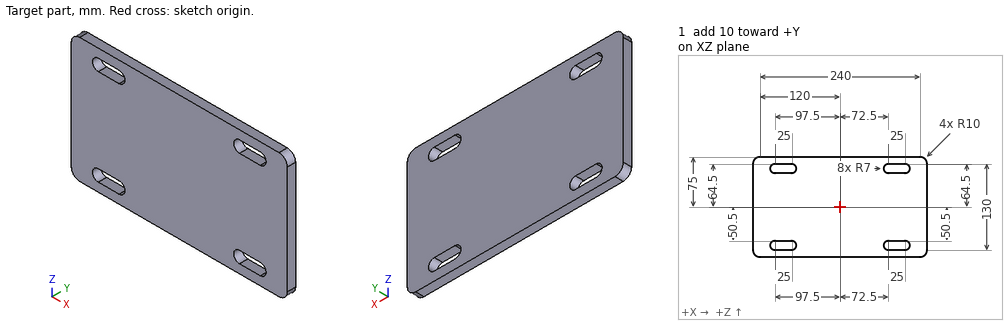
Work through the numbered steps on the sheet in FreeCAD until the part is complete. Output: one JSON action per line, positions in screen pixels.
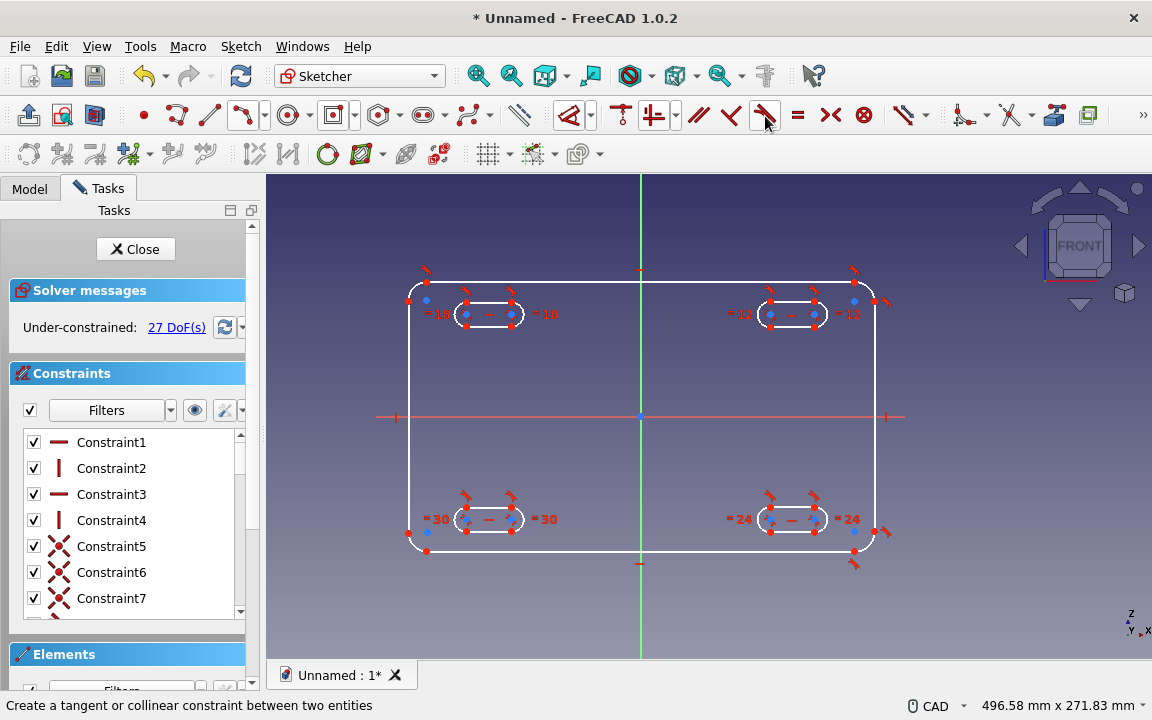
{"action": "left_click", "coordinate": [726, 552]}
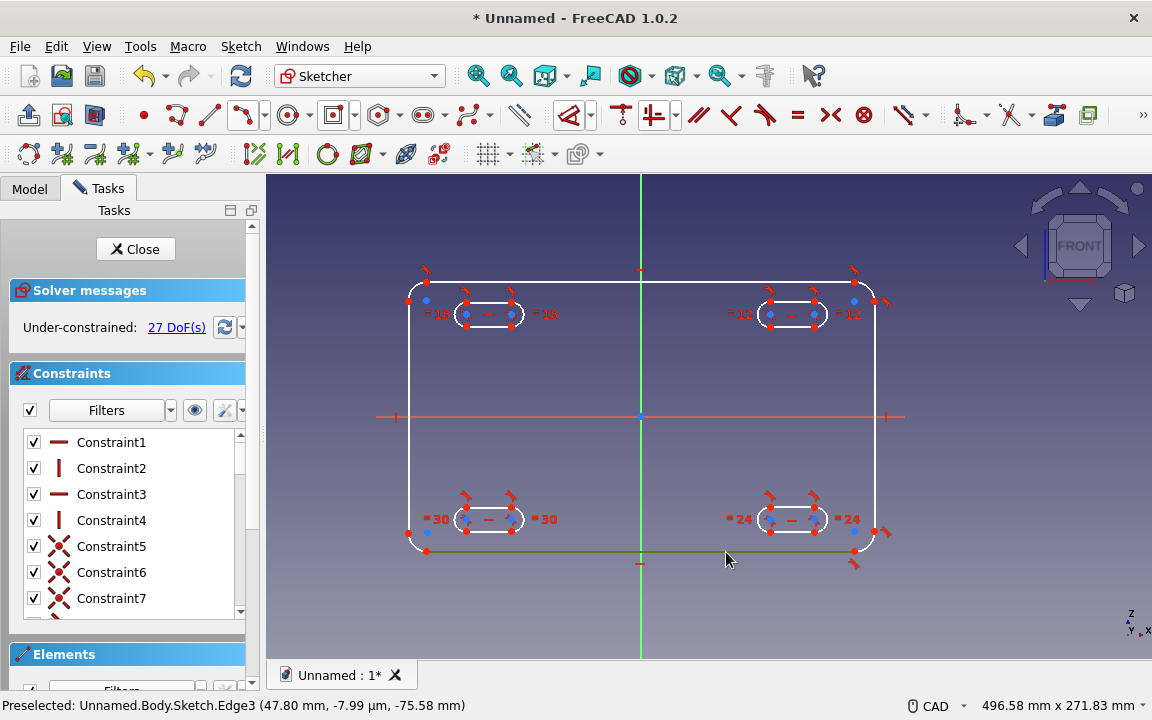
{"action": "left_click", "coordinate": [414, 546]}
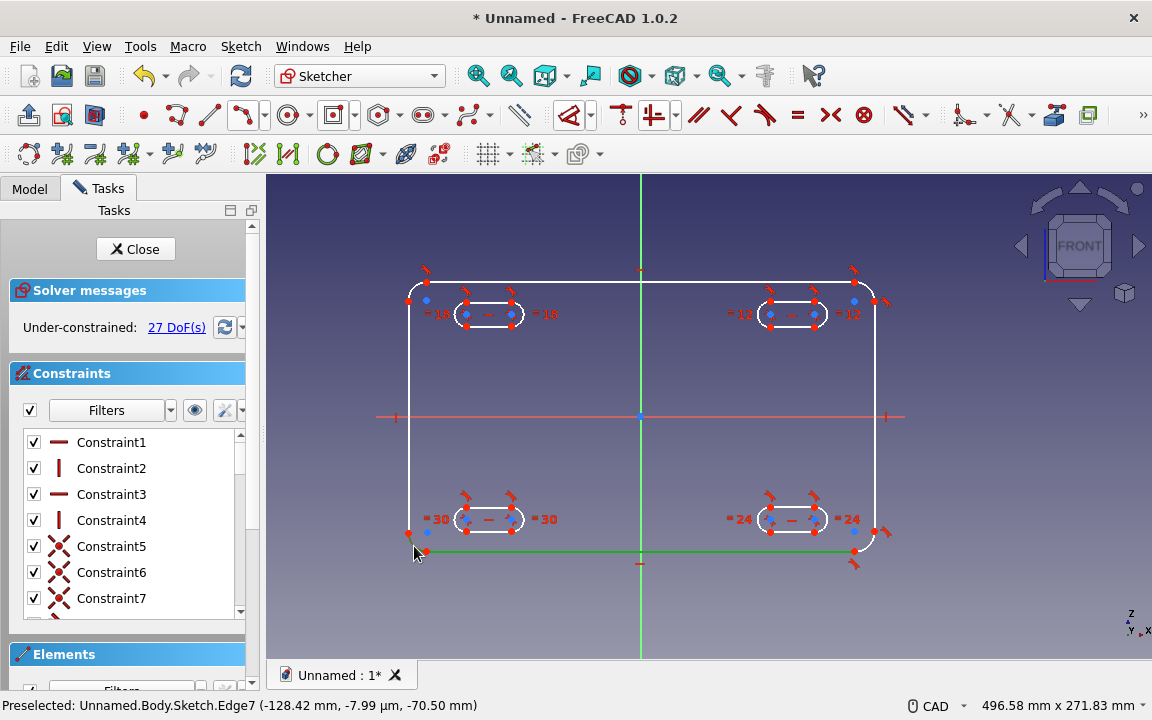
{"action": "left_click", "coordinate": [765, 116]}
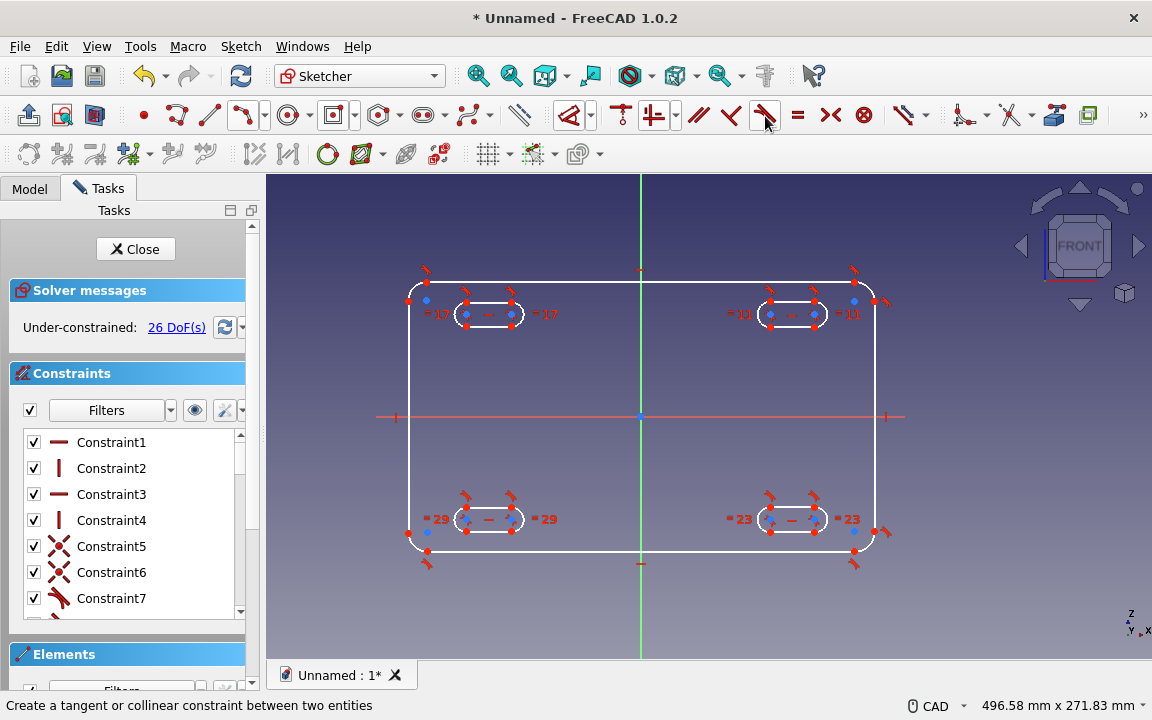
{"action": "left_click", "coordinate": [409, 464]}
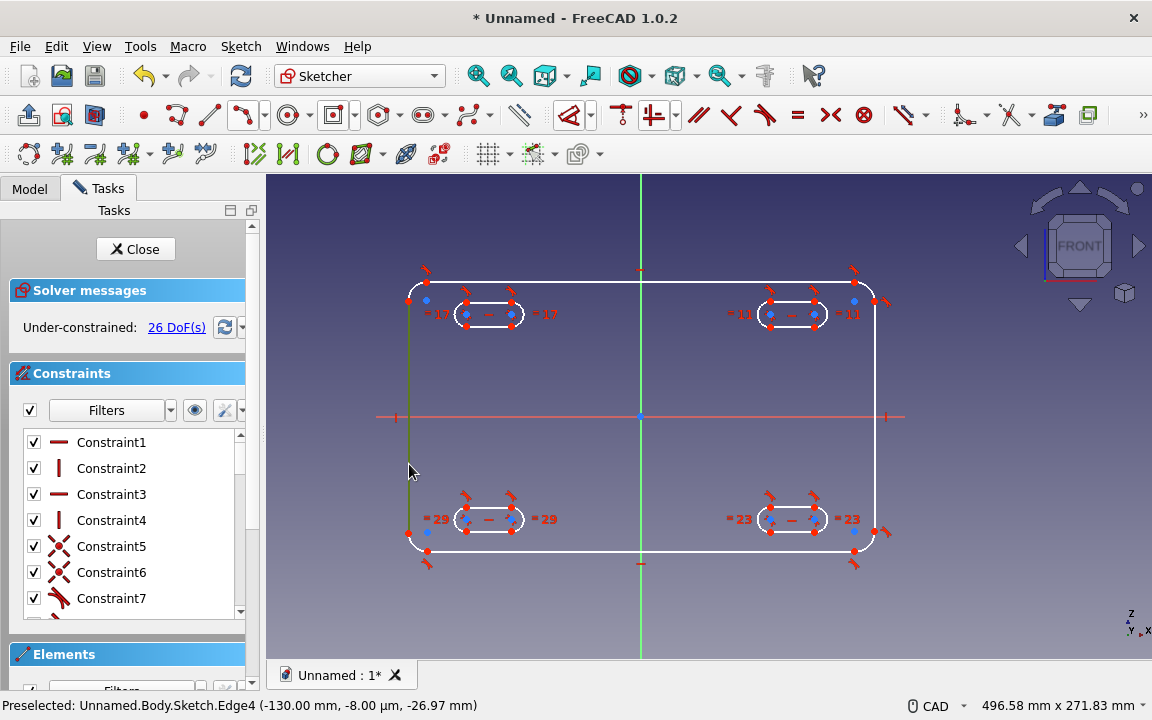
{"action": "left_click", "coordinate": [415, 547]}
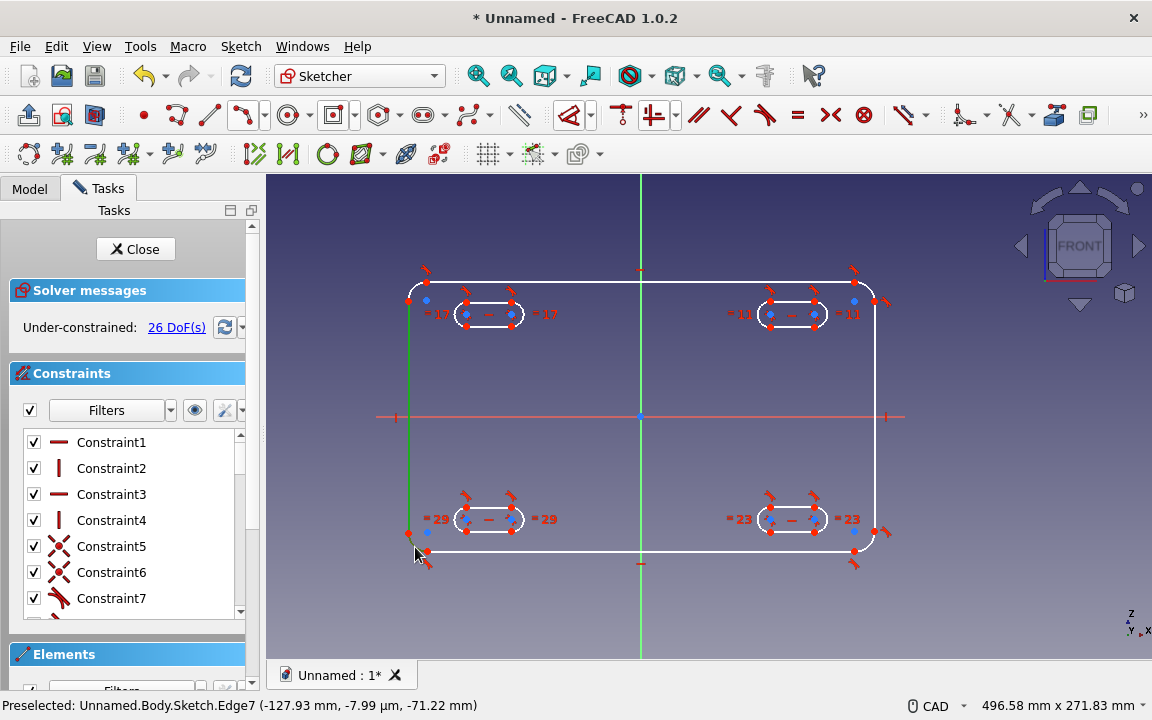
{"action": "left_click", "coordinate": [765, 116]}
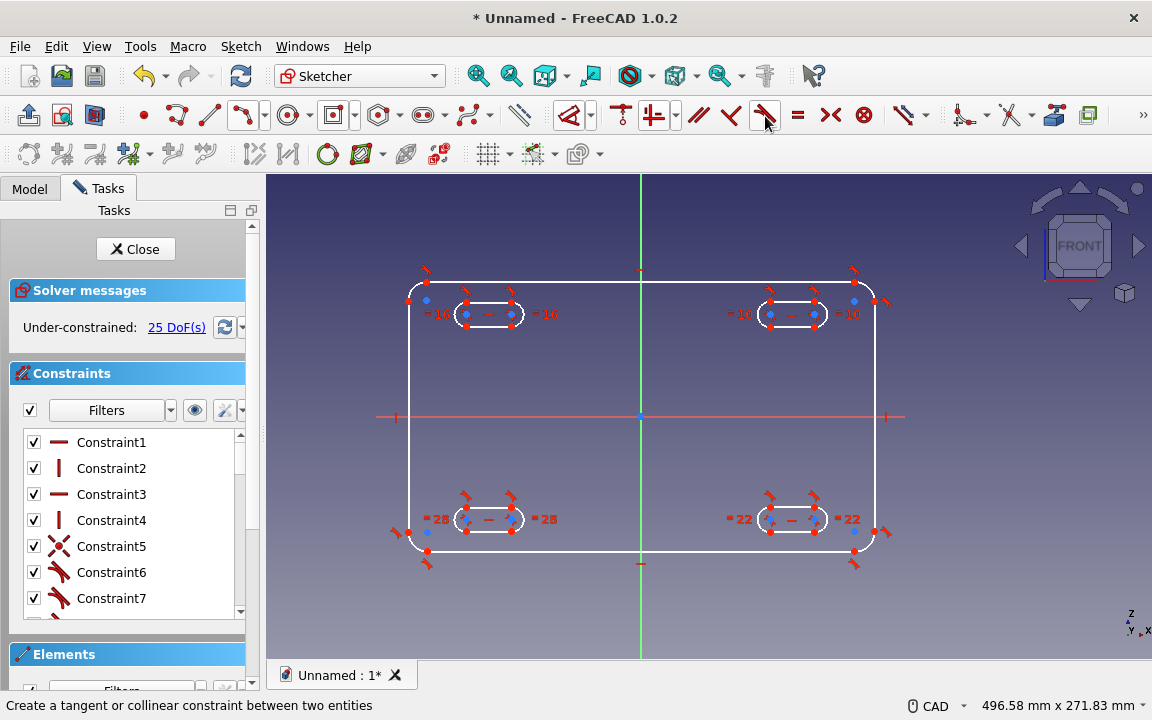
{"action": "left_click", "coordinate": [409, 463]}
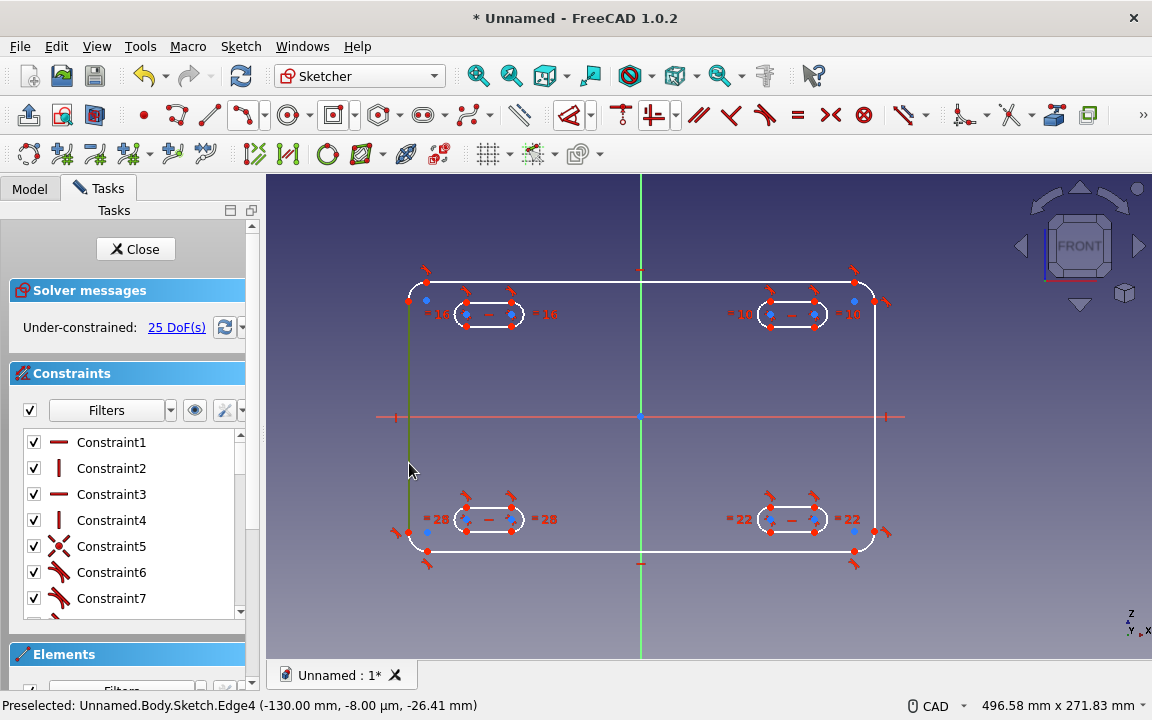
{"action": "left_click", "coordinate": [413, 288]}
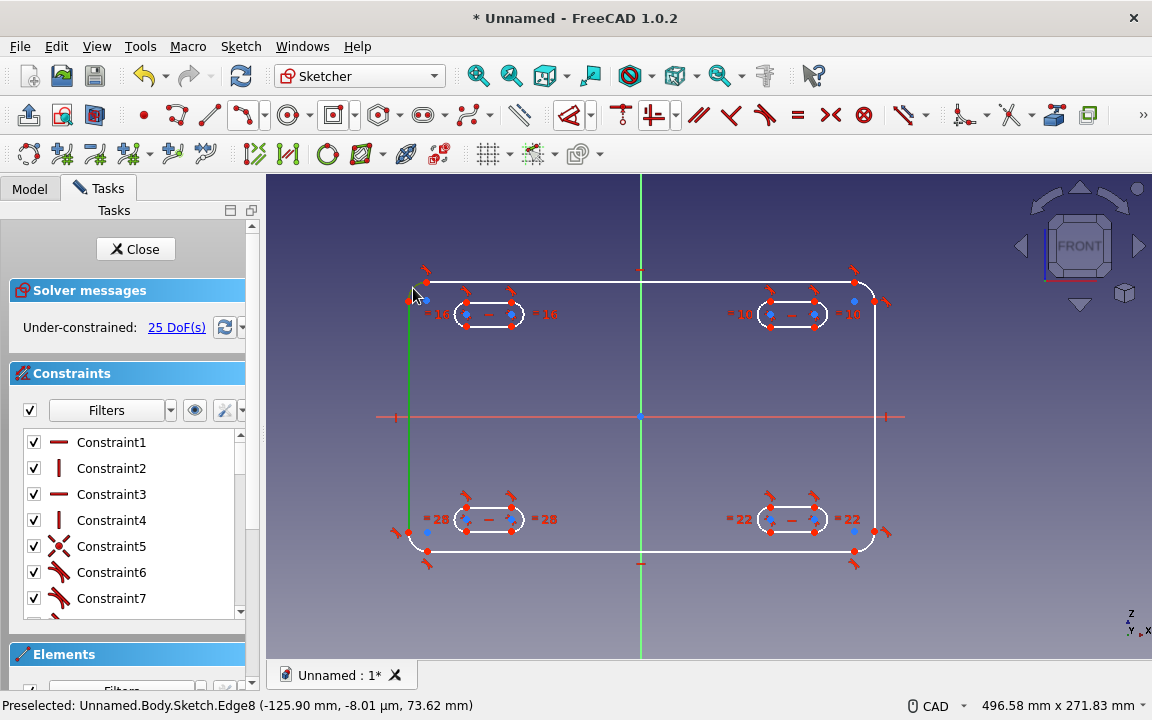
{"action": "left_click", "coordinate": [765, 116]}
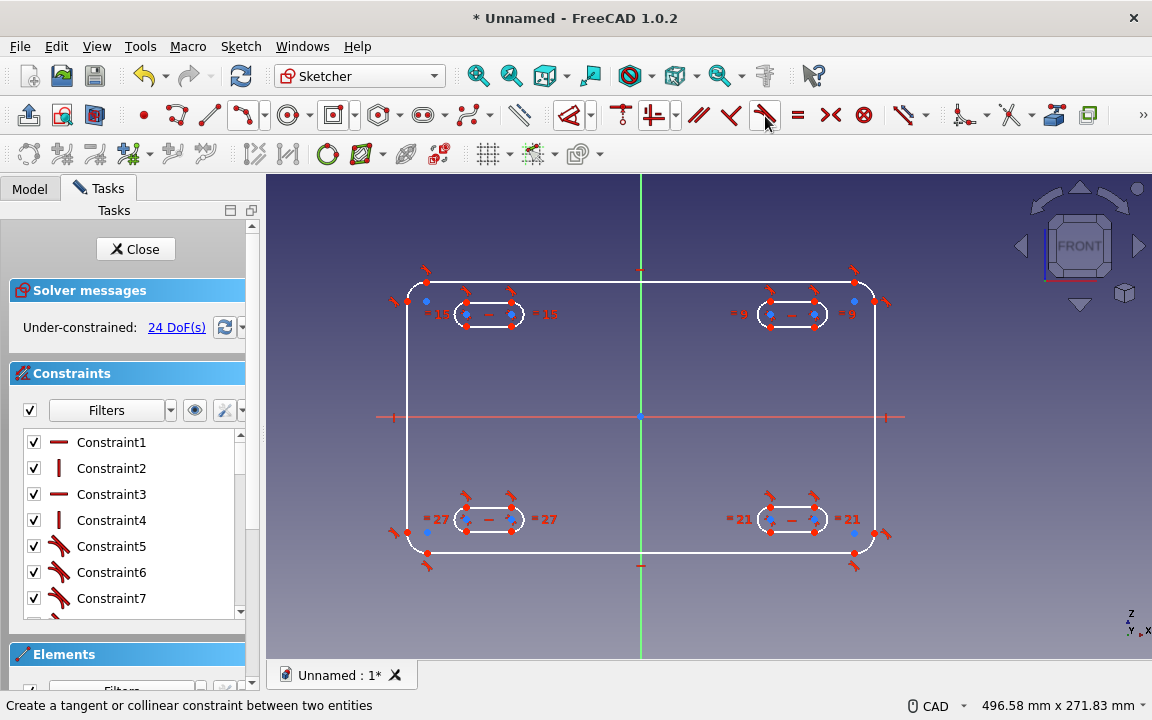
{"action": "scroll", "coordinate": [872, 293], "scroll_direction": "up", "scroll_amount": 3}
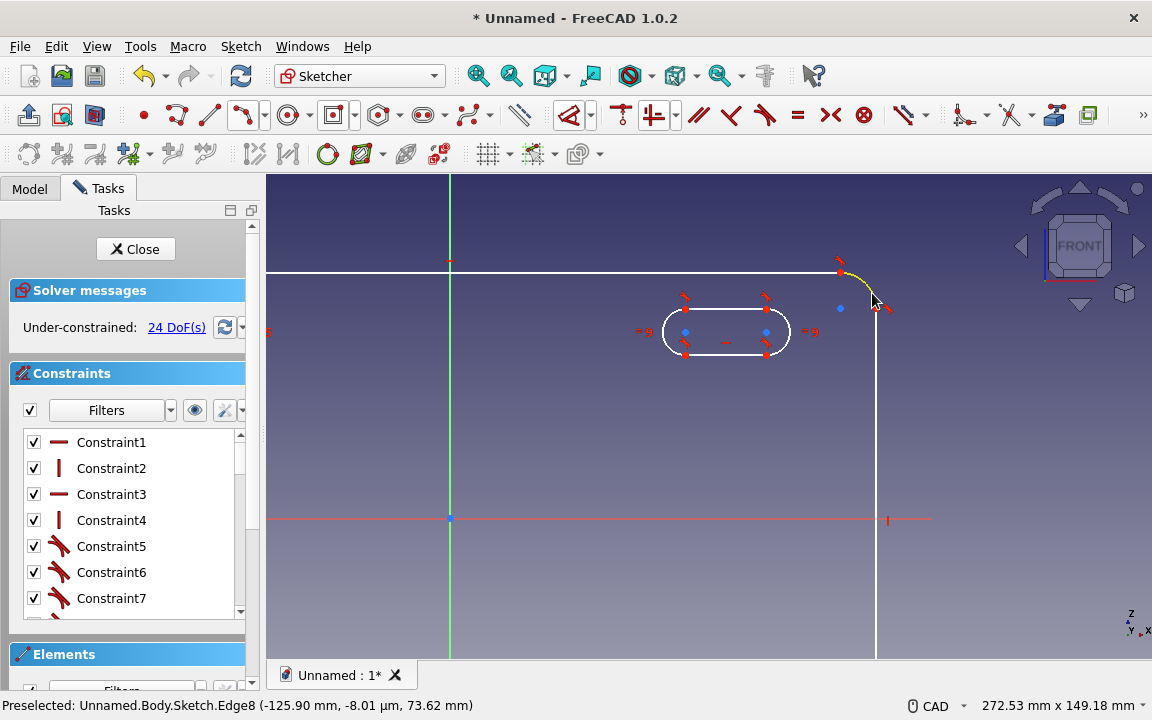
{"action": "left_click", "coordinate": [872, 293]}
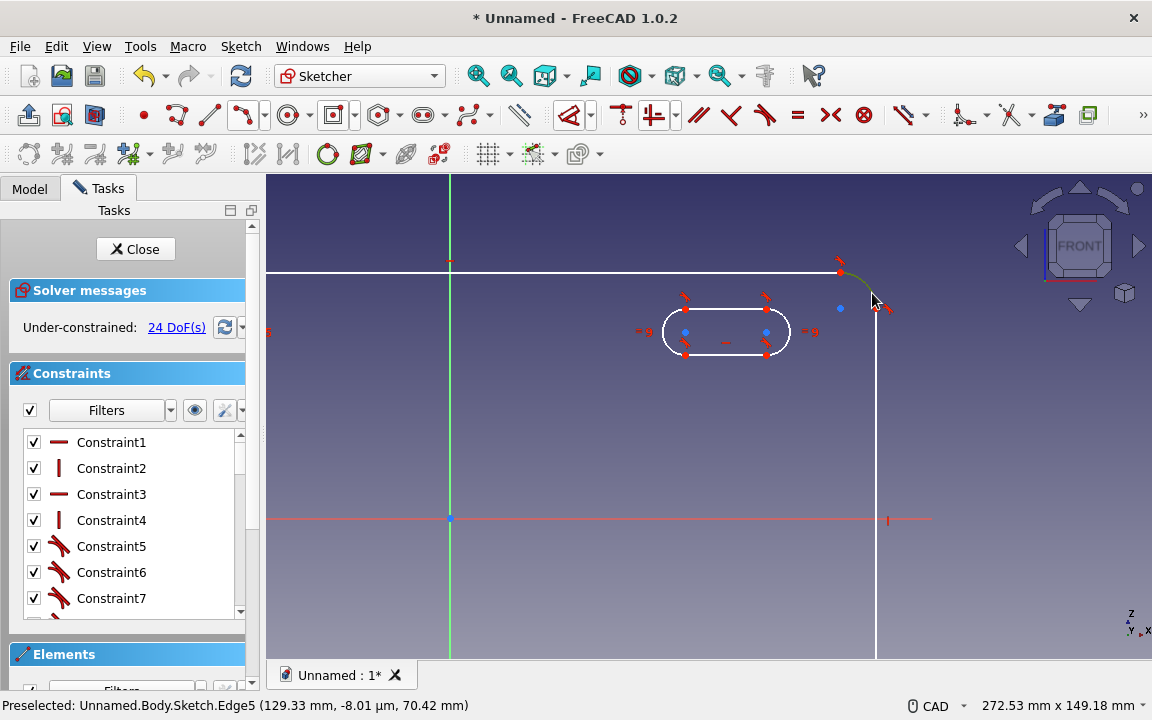
{"action": "scroll", "coordinate": [872, 292], "scroll_direction": "down", "scroll_amount": 3}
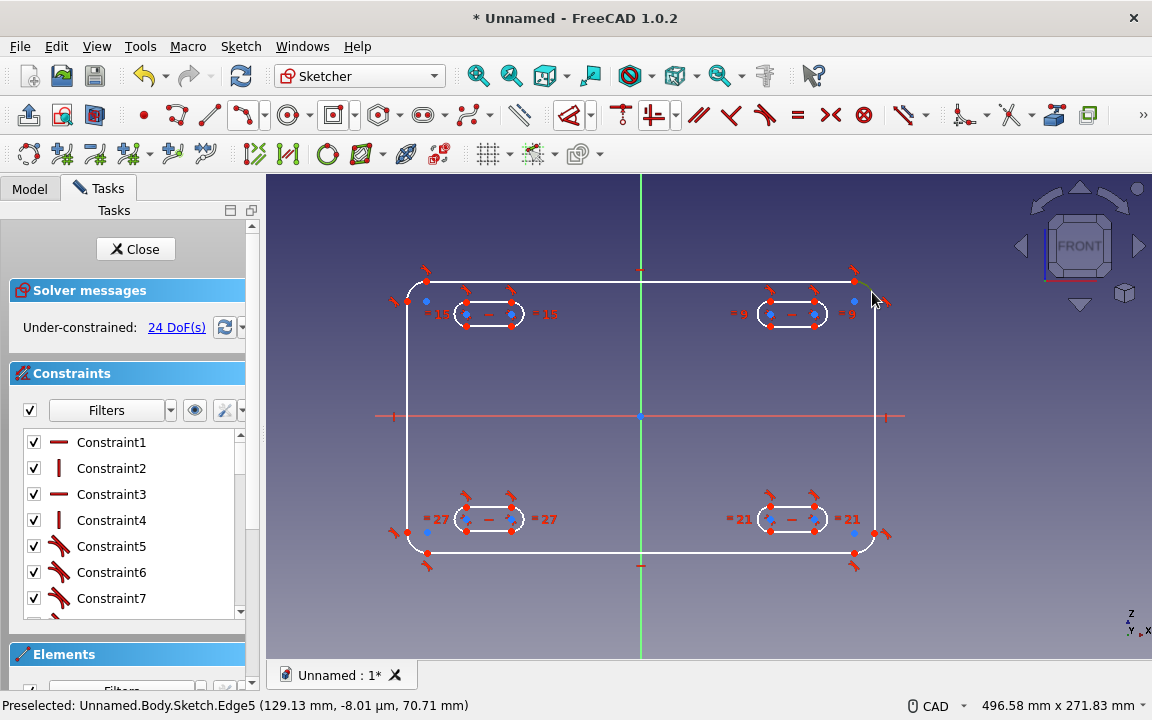
{"action": "scroll", "coordinate": [864, 551], "scroll_direction": "up", "scroll_amount": 3}